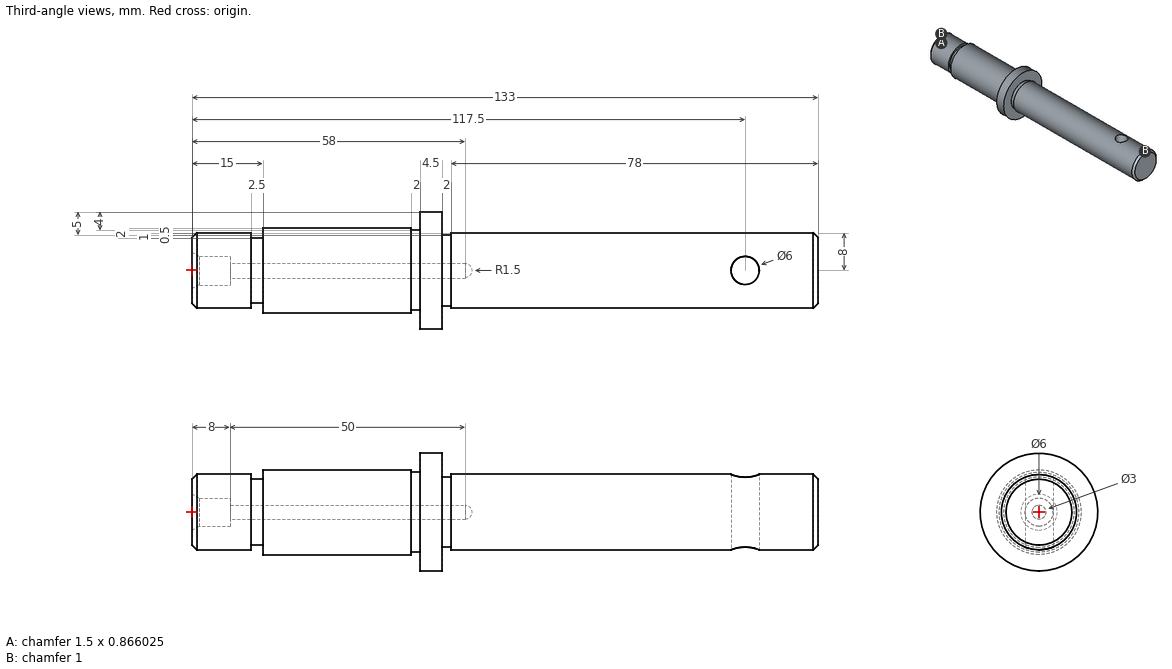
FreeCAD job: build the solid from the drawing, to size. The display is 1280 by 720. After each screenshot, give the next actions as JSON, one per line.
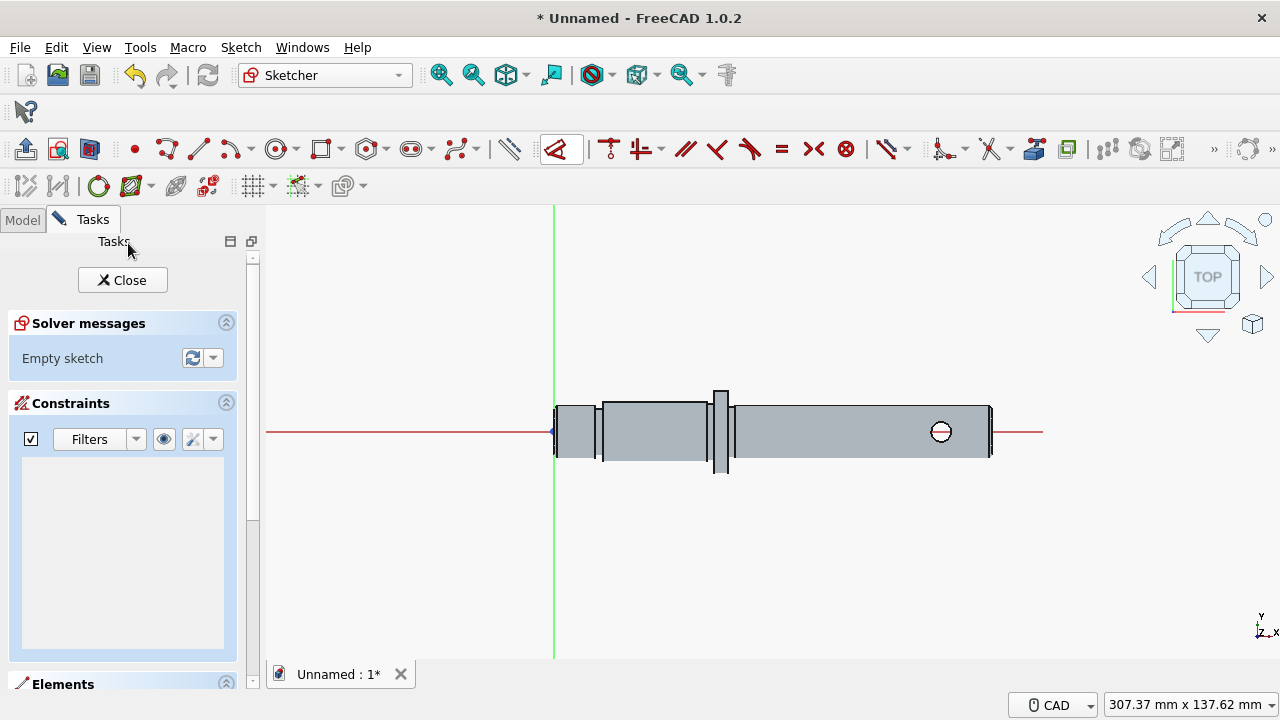
{"action": "key", "text": "q s"}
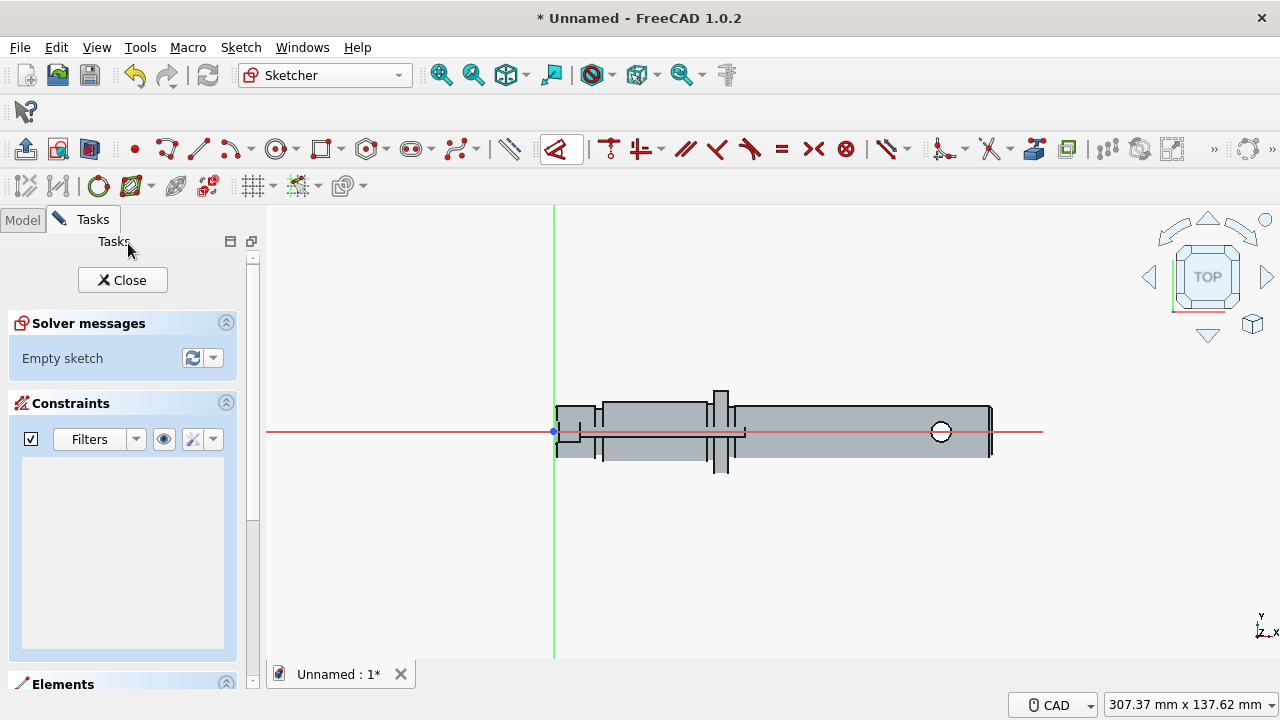
{"action": "scroll", "coordinate": [750, 434], "scroll_direction": "up", "scroll_amount": 15}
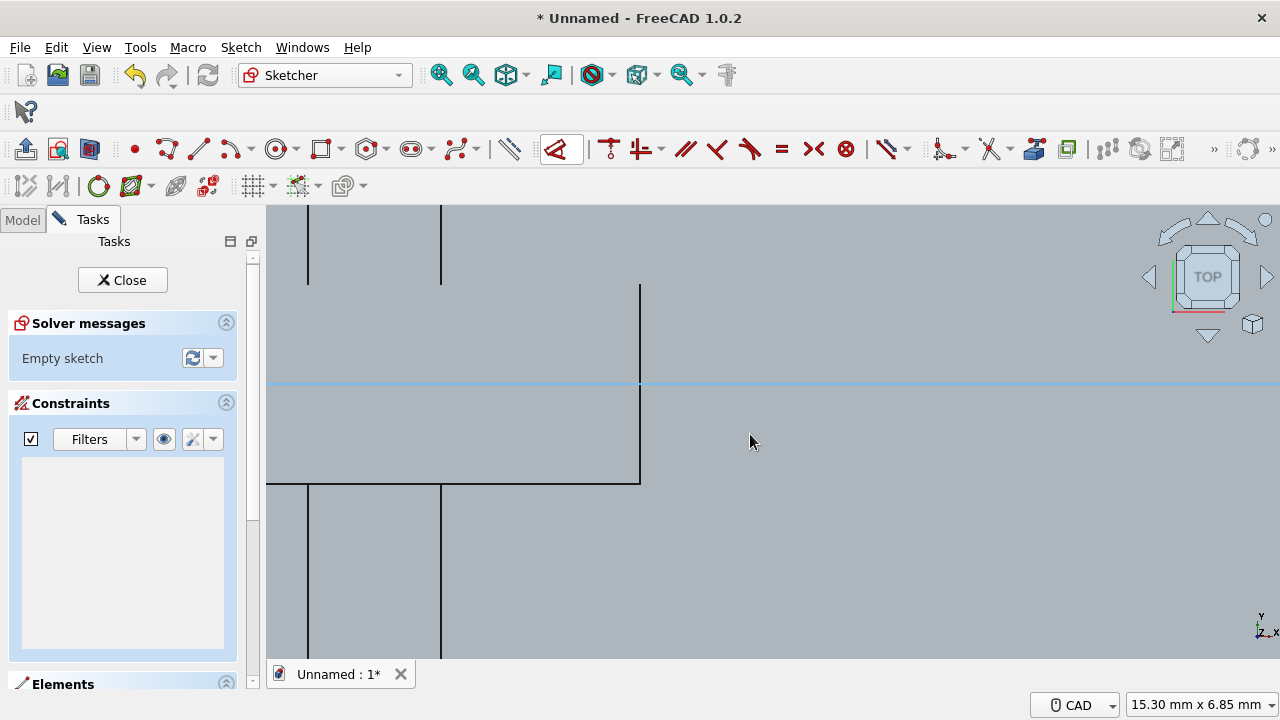
{"action": "left_click", "coordinate": [200, 150]}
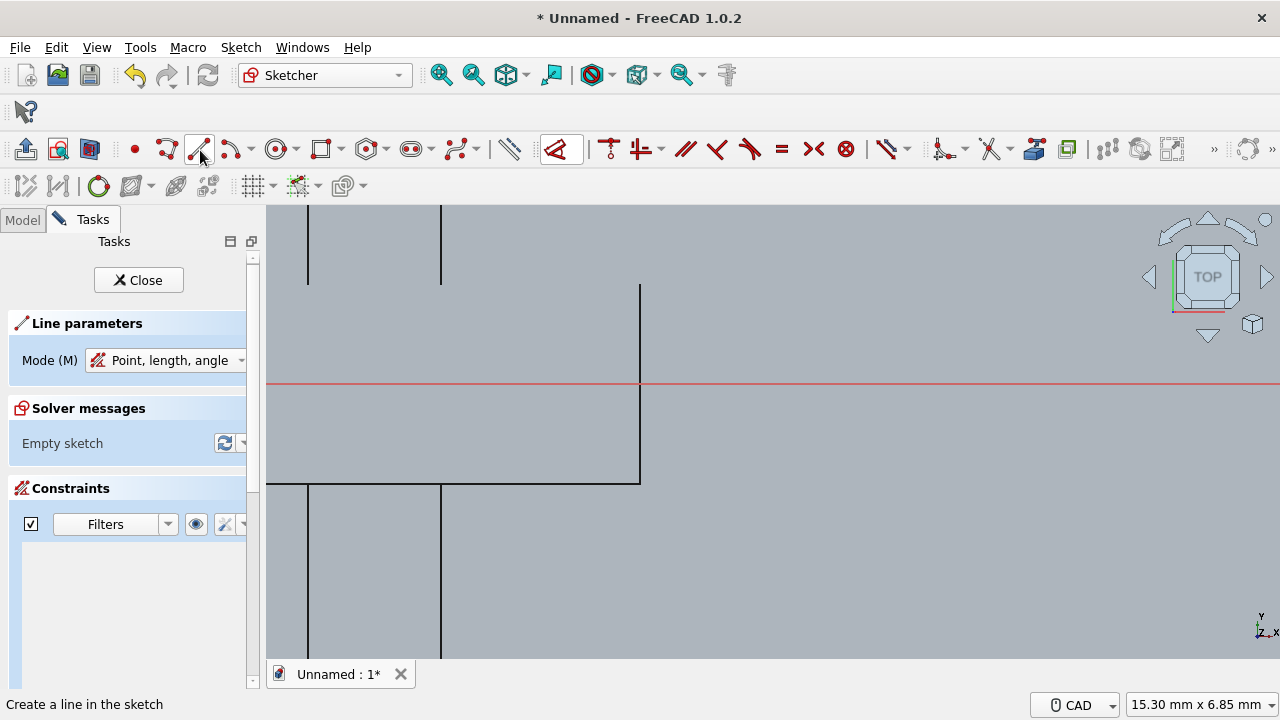
{"action": "left_click", "coordinate": [640, 285]}
{"action": "left_click", "coordinate": [640, 484]}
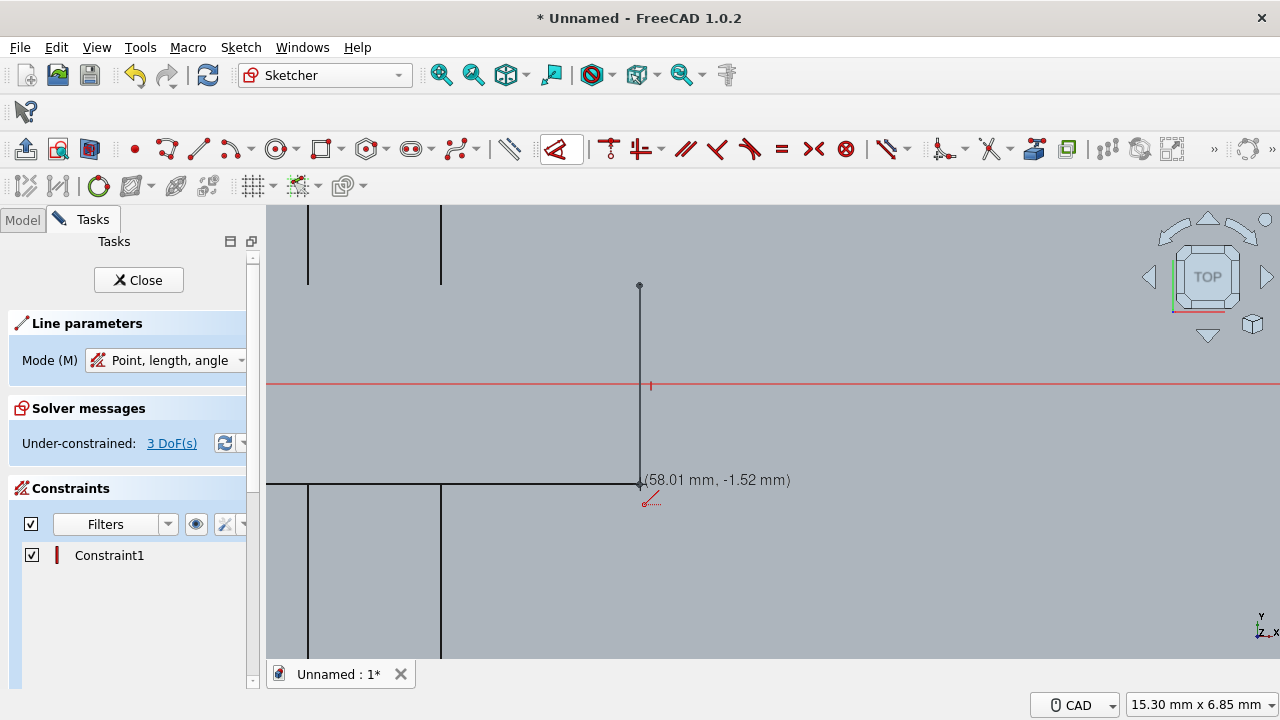
{"action": "left_click", "coordinate": [254, 150]}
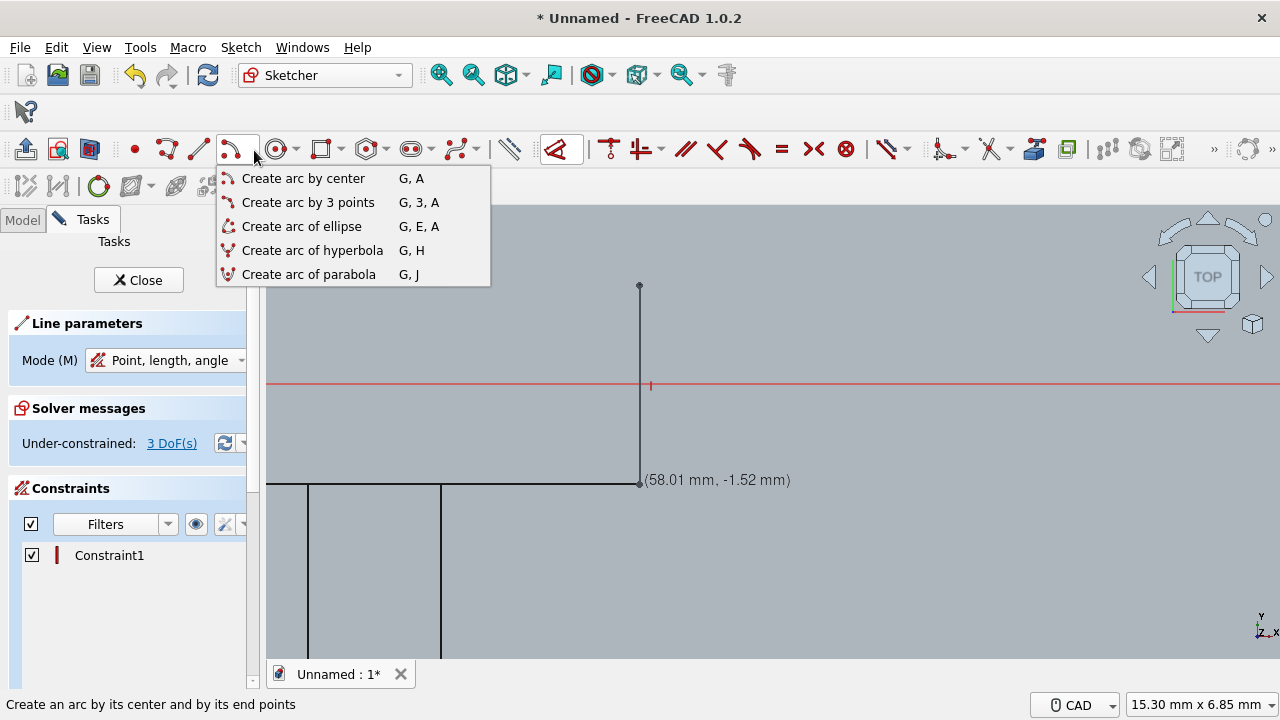
{"action": "left_click", "coordinate": [354, 202]}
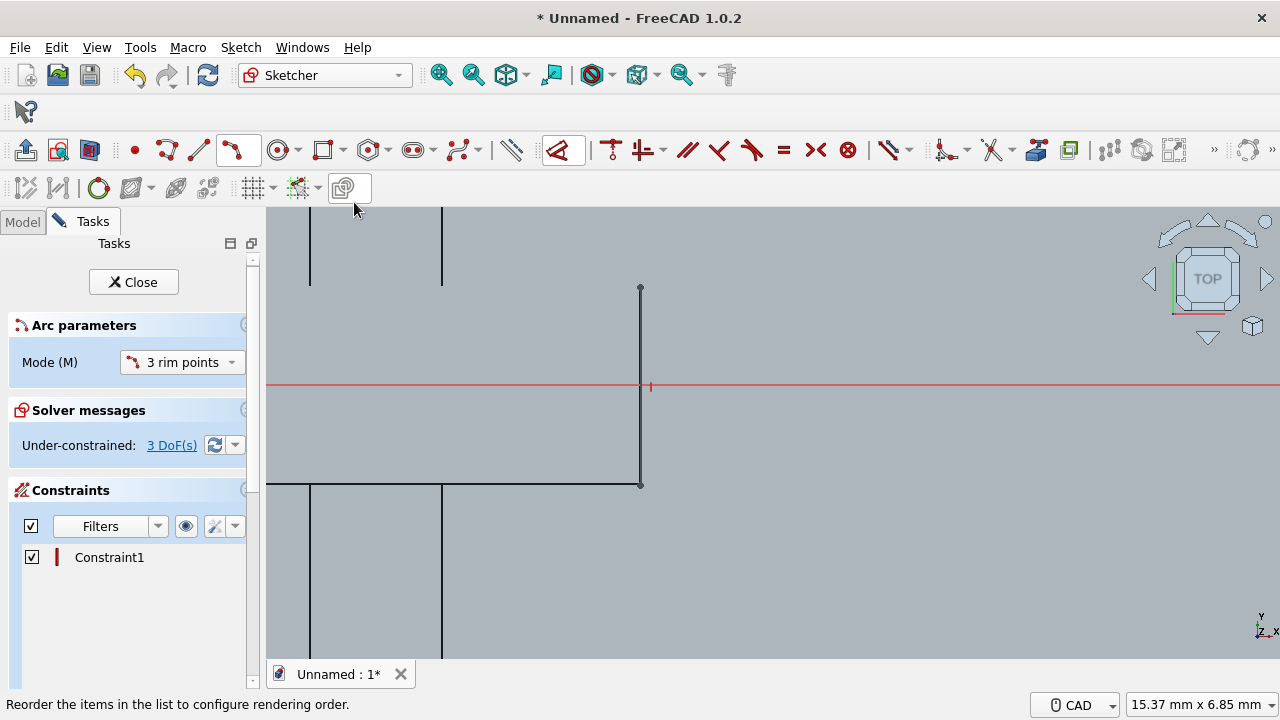
{"action": "left_click", "coordinate": [641, 486]}
{"action": "left_click", "coordinate": [641, 288]}
{"action": "left_click", "coordinate": [734, 416]}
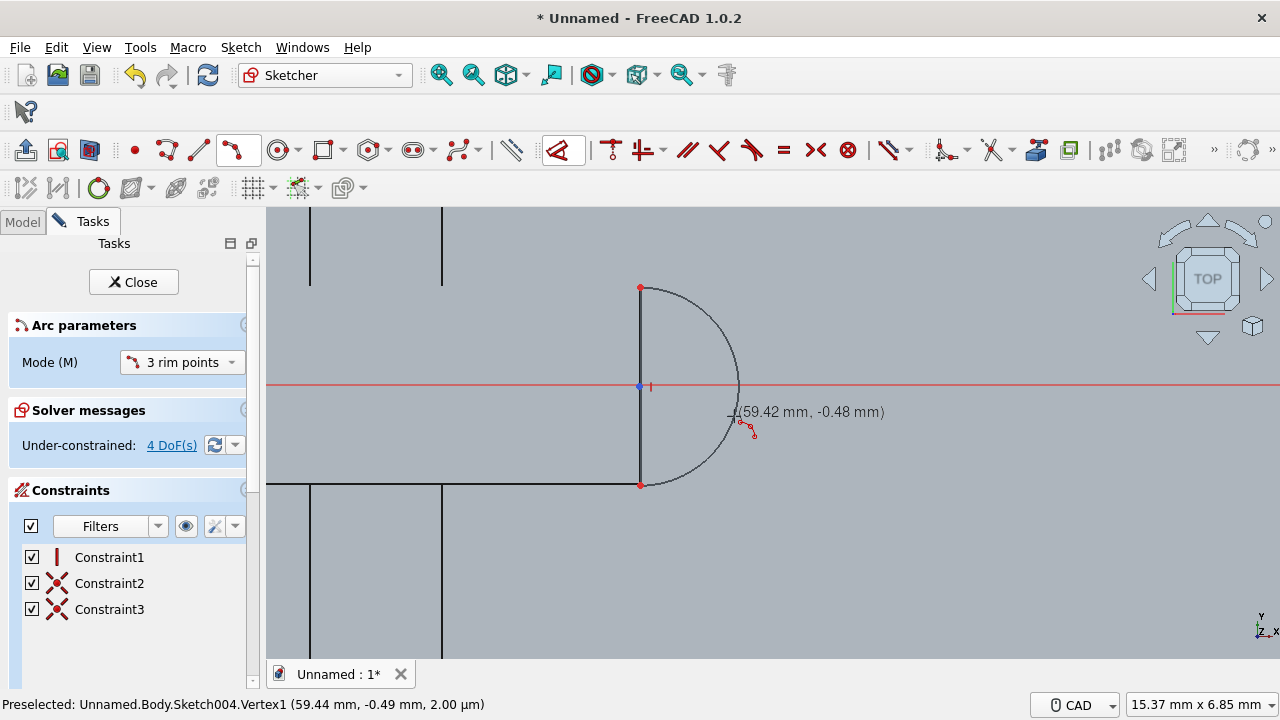
{"action": "left_click", "coordinate": [200, 150]}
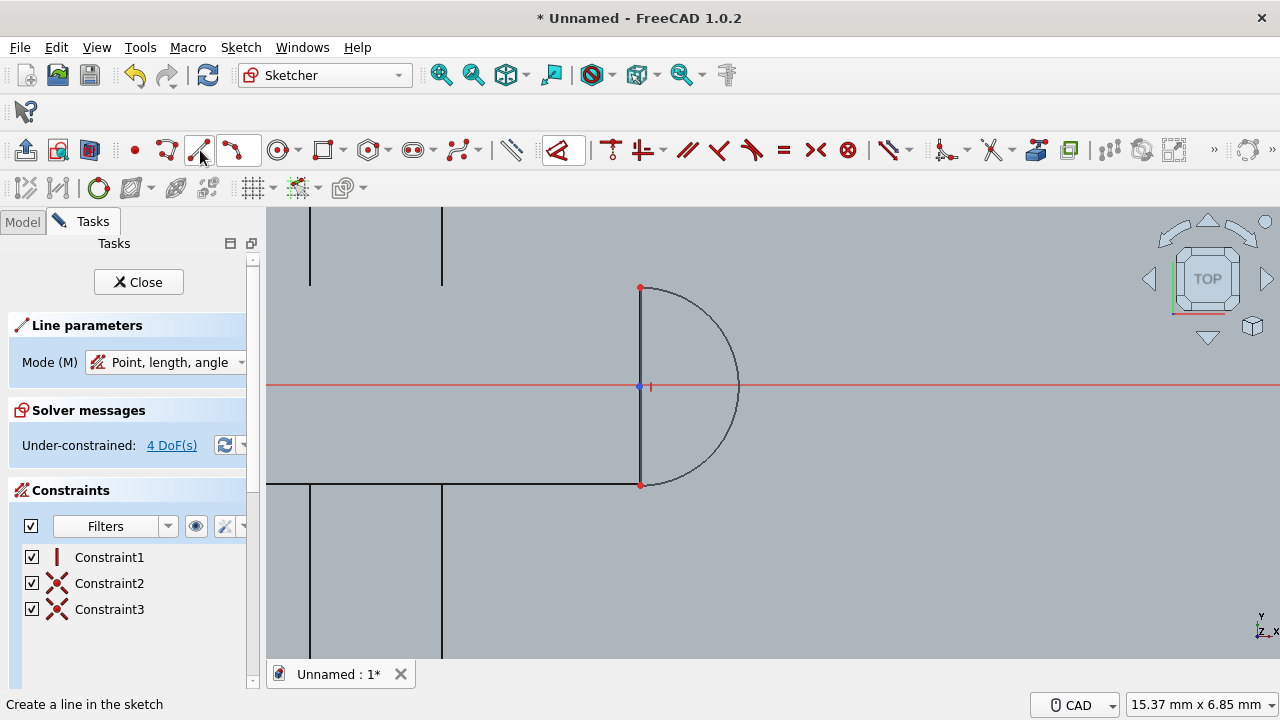
{"action": "left_click", "coordinate": [640, 504]}
{"action": "left_click", "coordinate": [640, 564]}
{"action": "key", "text": "Escape"}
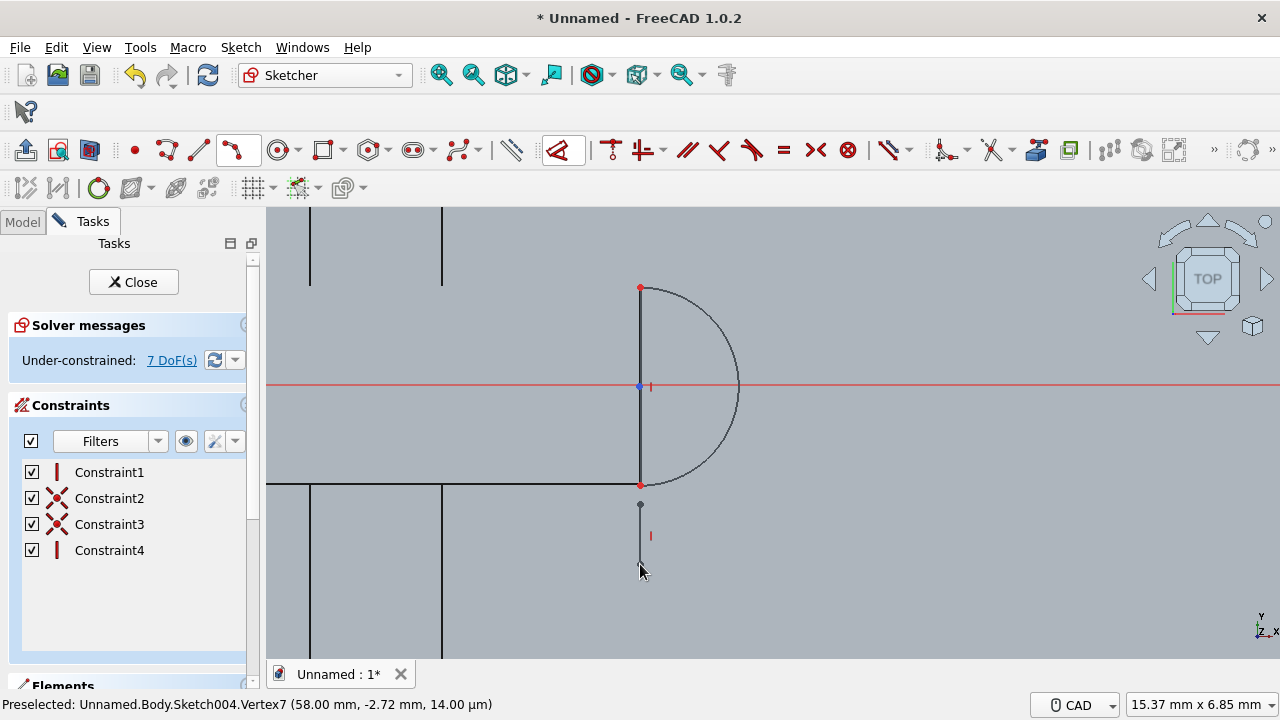
{"action": "left_click", "coordinate": [640, 523]}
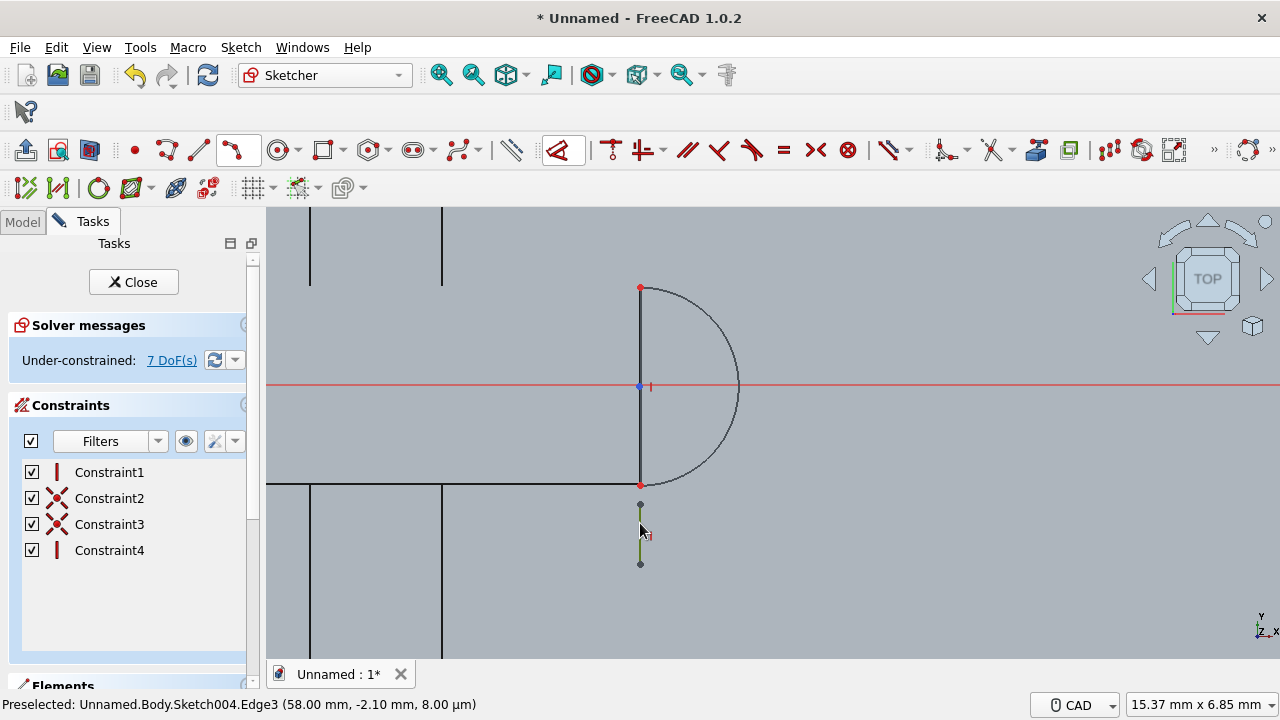
{"action": "left_click", "coordinate": [512, 150]}